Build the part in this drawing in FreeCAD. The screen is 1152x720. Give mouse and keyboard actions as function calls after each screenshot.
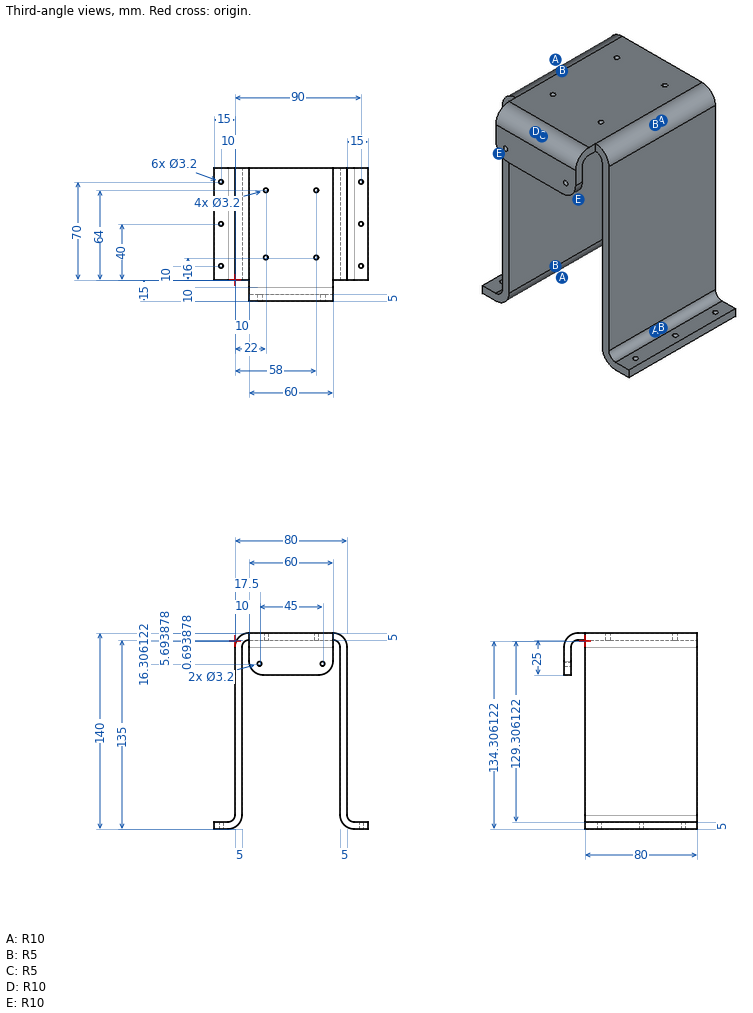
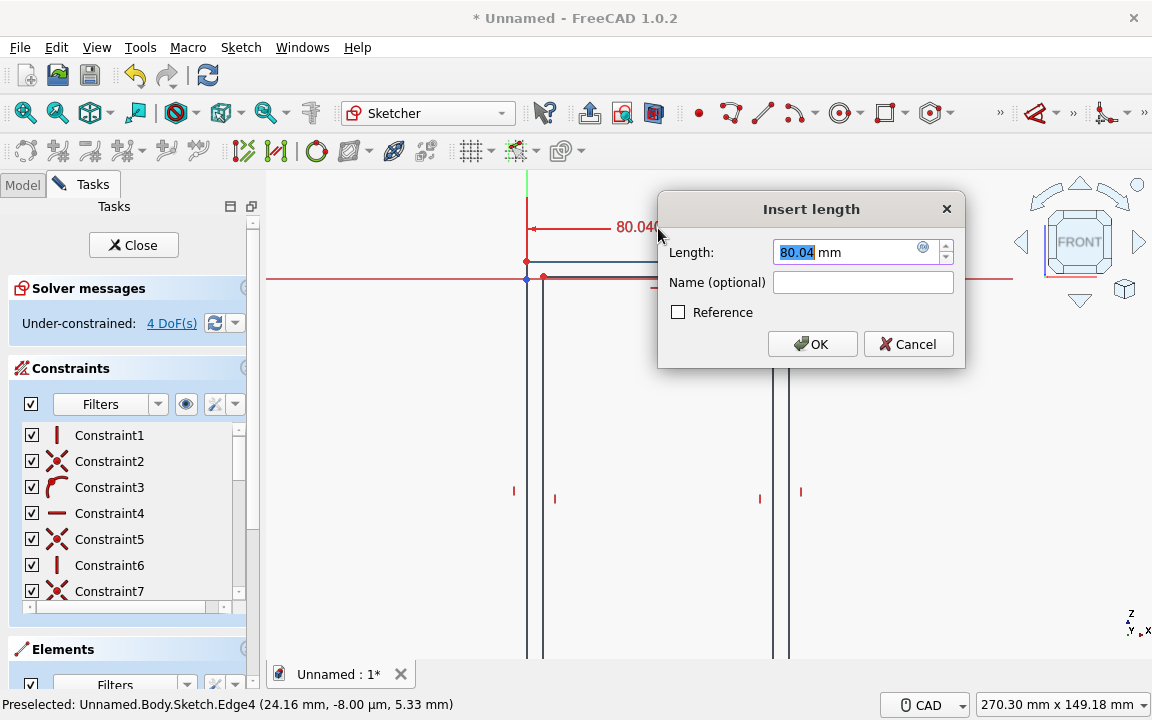
text(80)
key(Return)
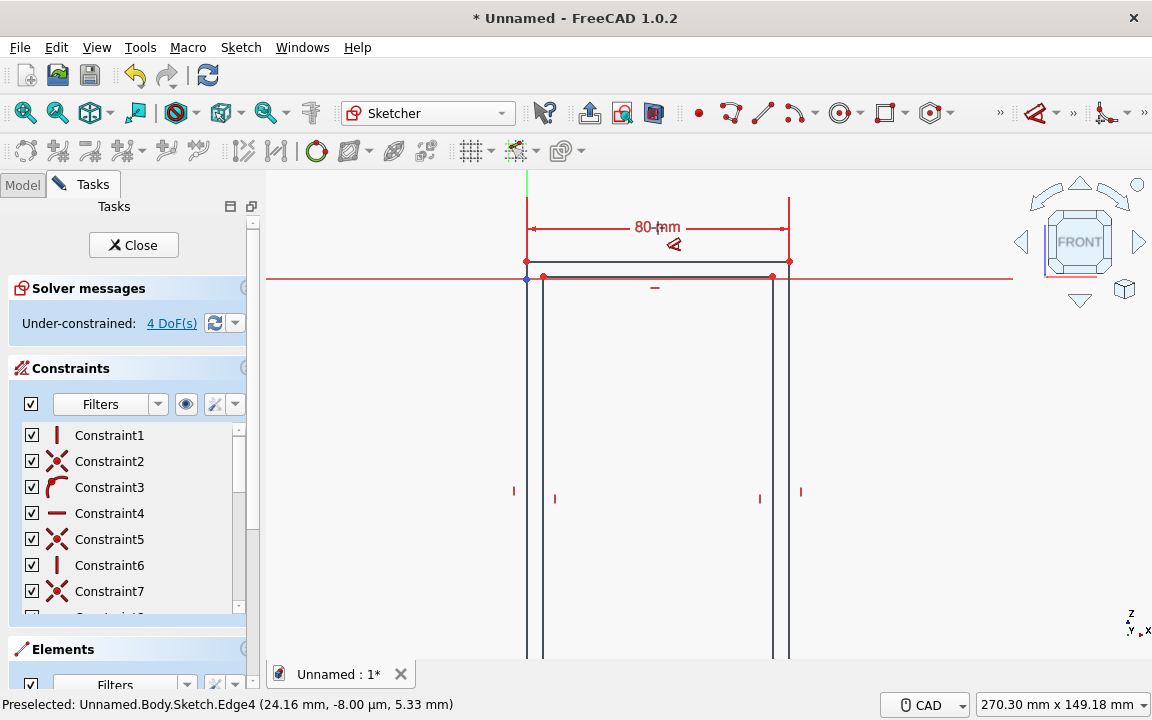
click(543, 410)
click(509, 454)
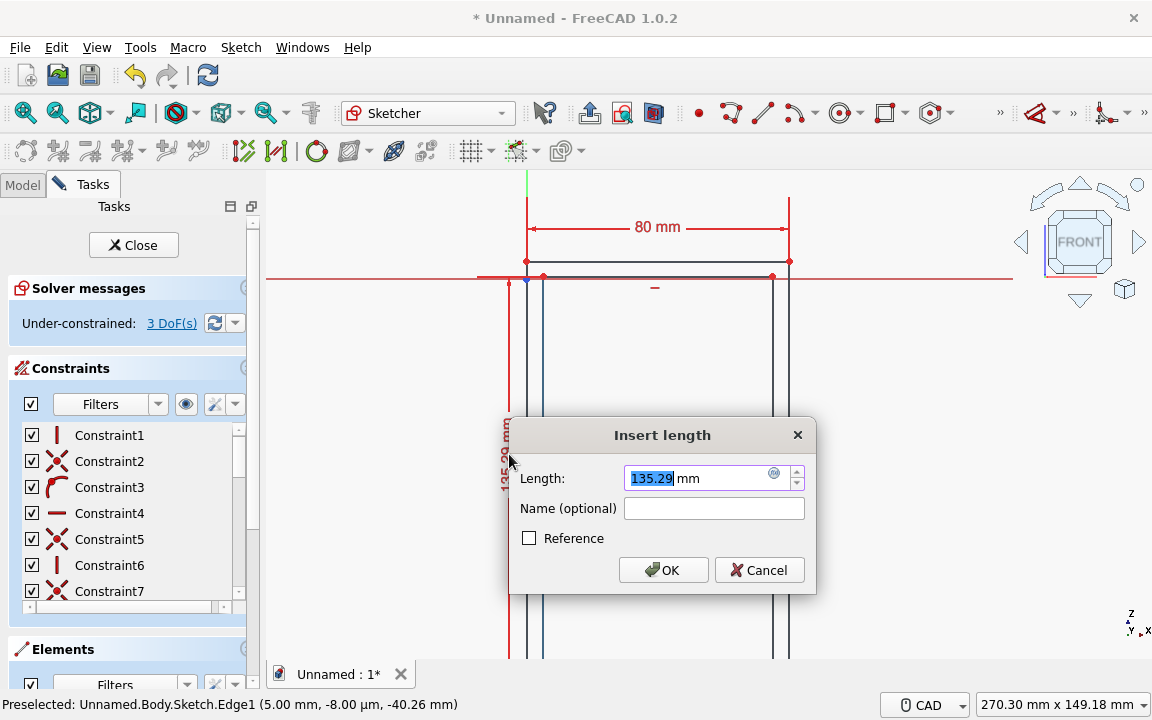
text(135)
key(Return)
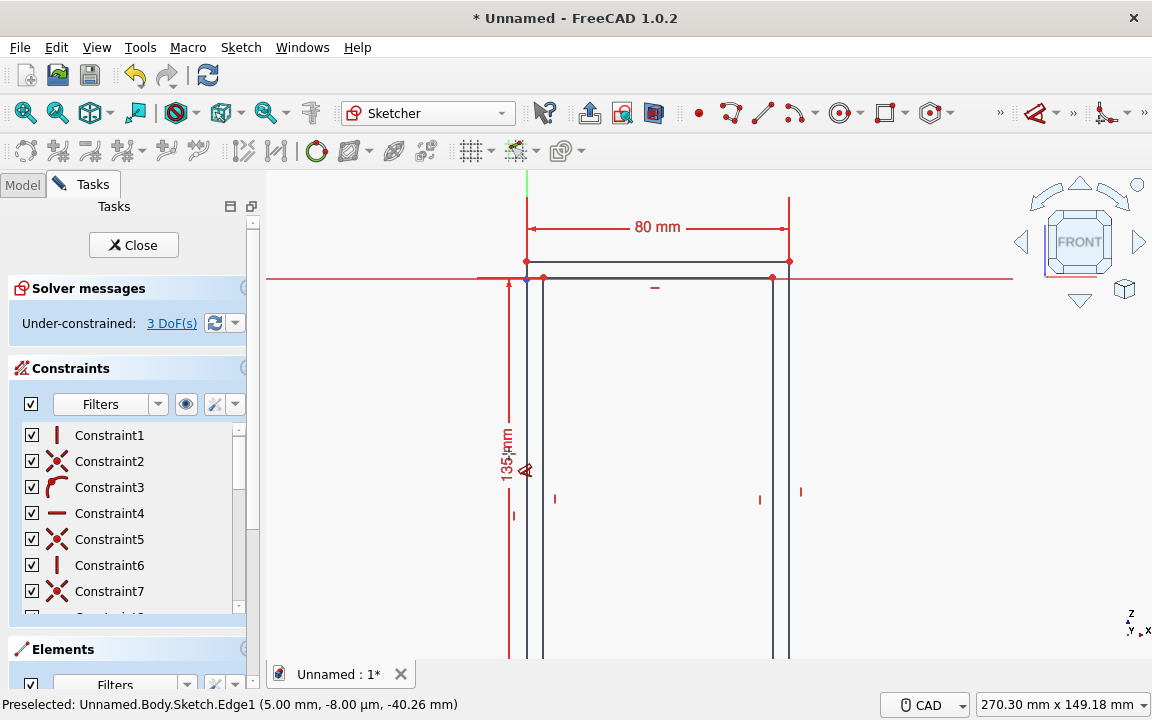
click(527, 583)
click(493, 361)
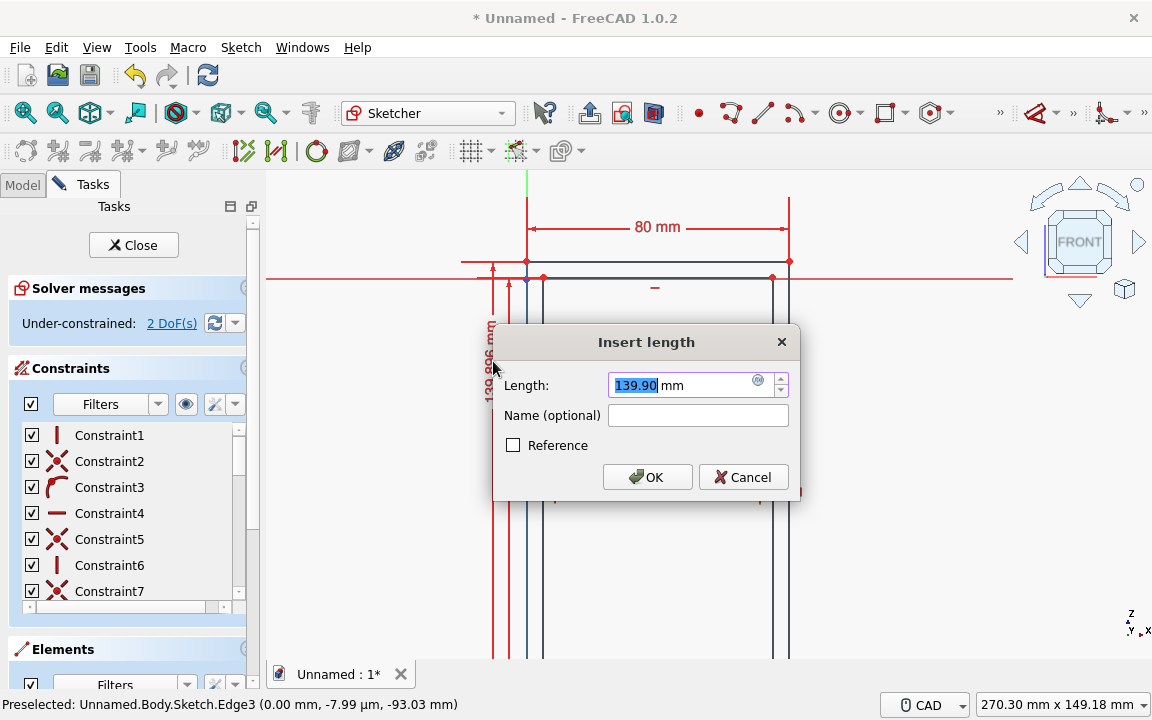
text(140)
key(Return)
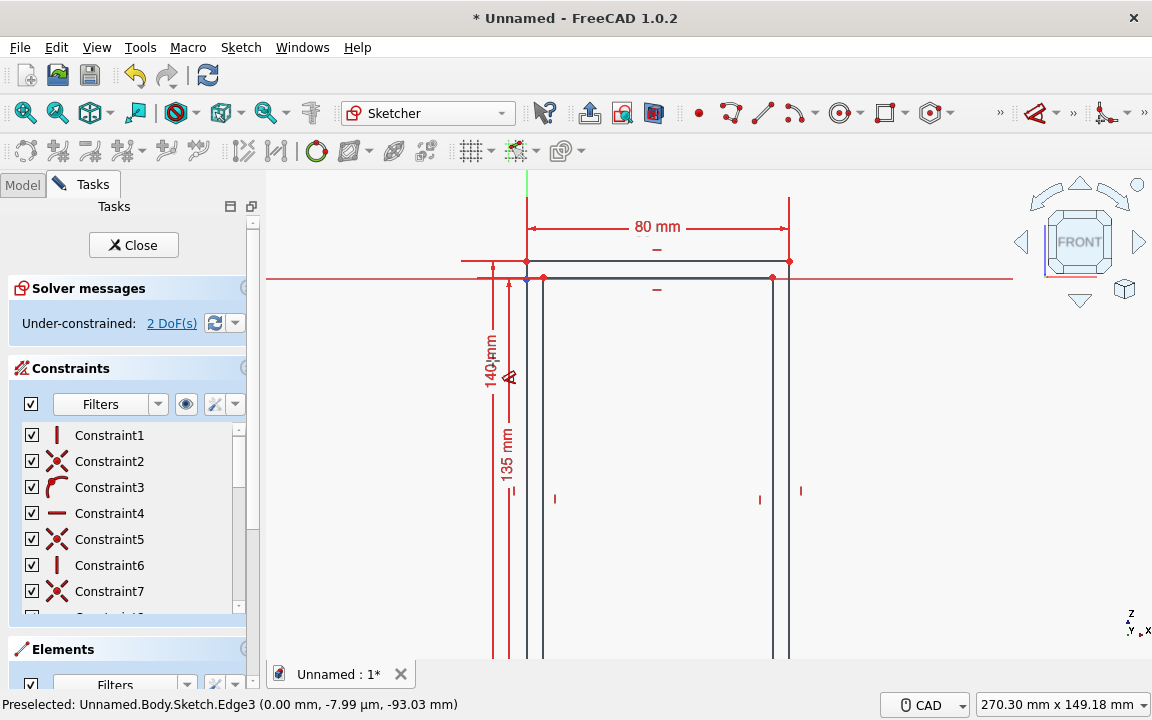
click(789, 399)
click(823, 446)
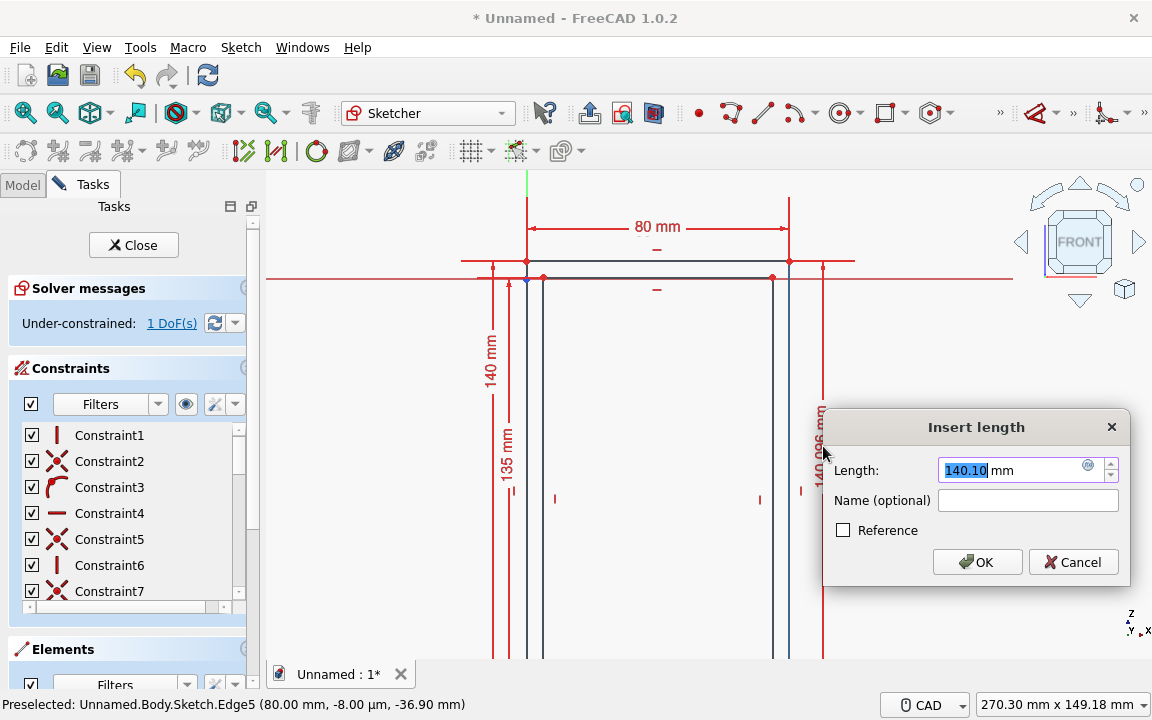
text(140)
key(Return)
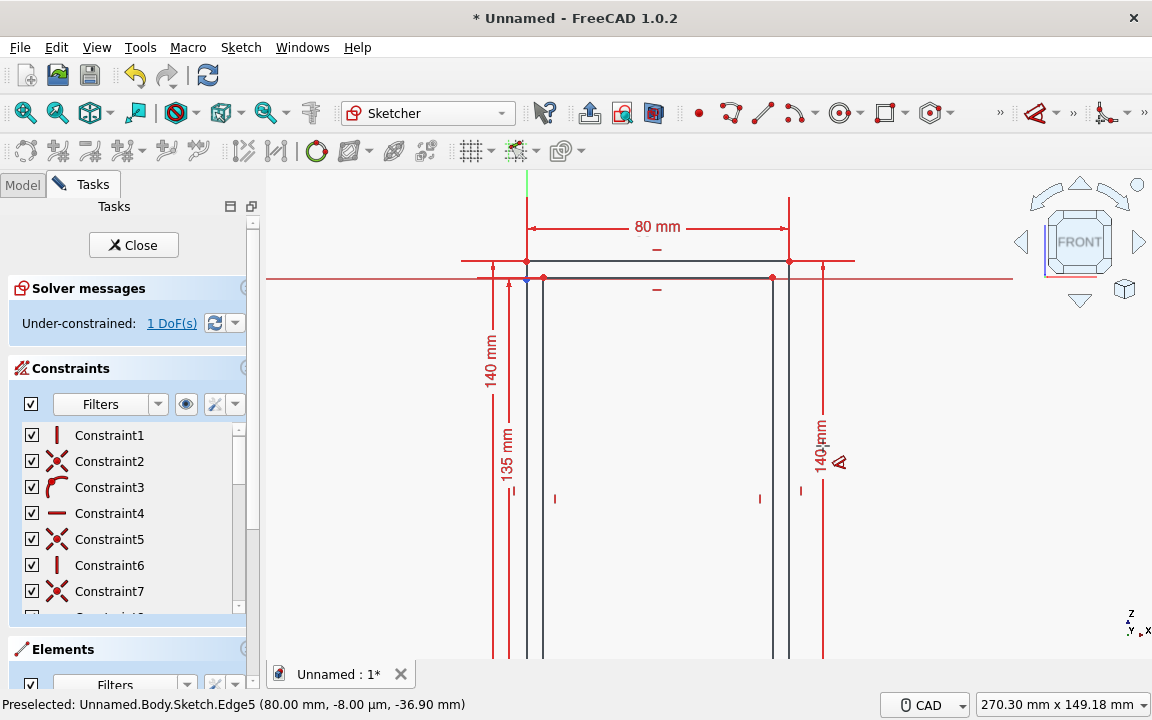
scroll(543, 278, up, 15)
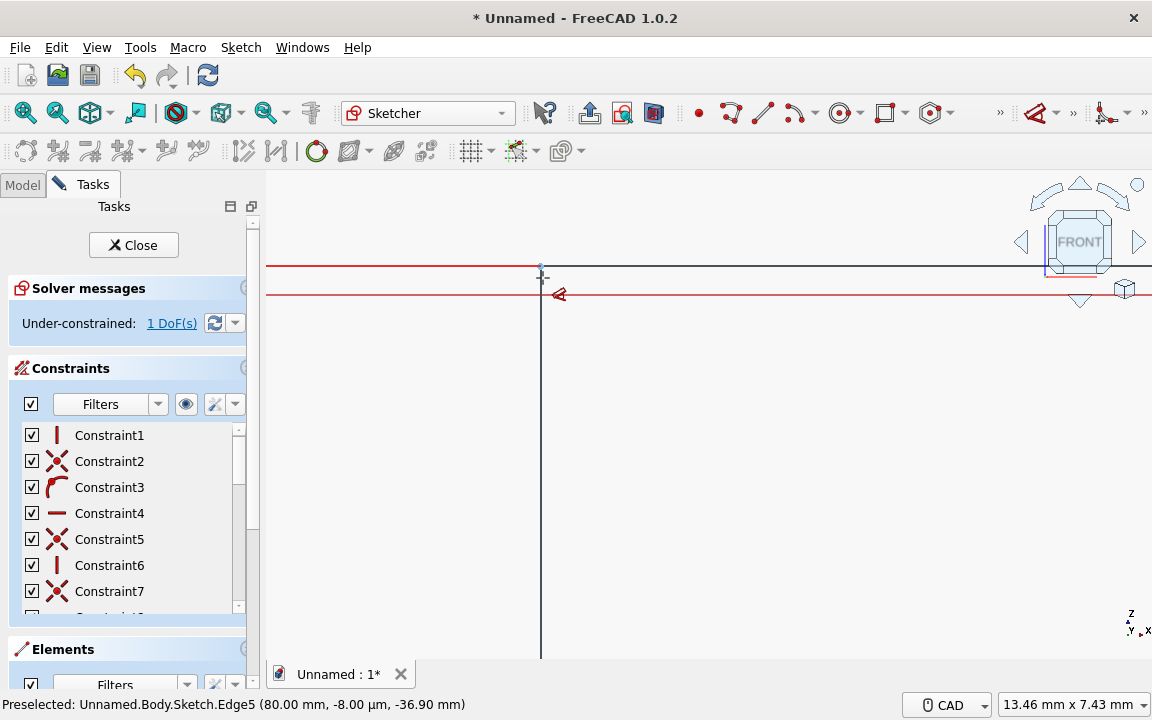
click(541, 266)
click(575, 281)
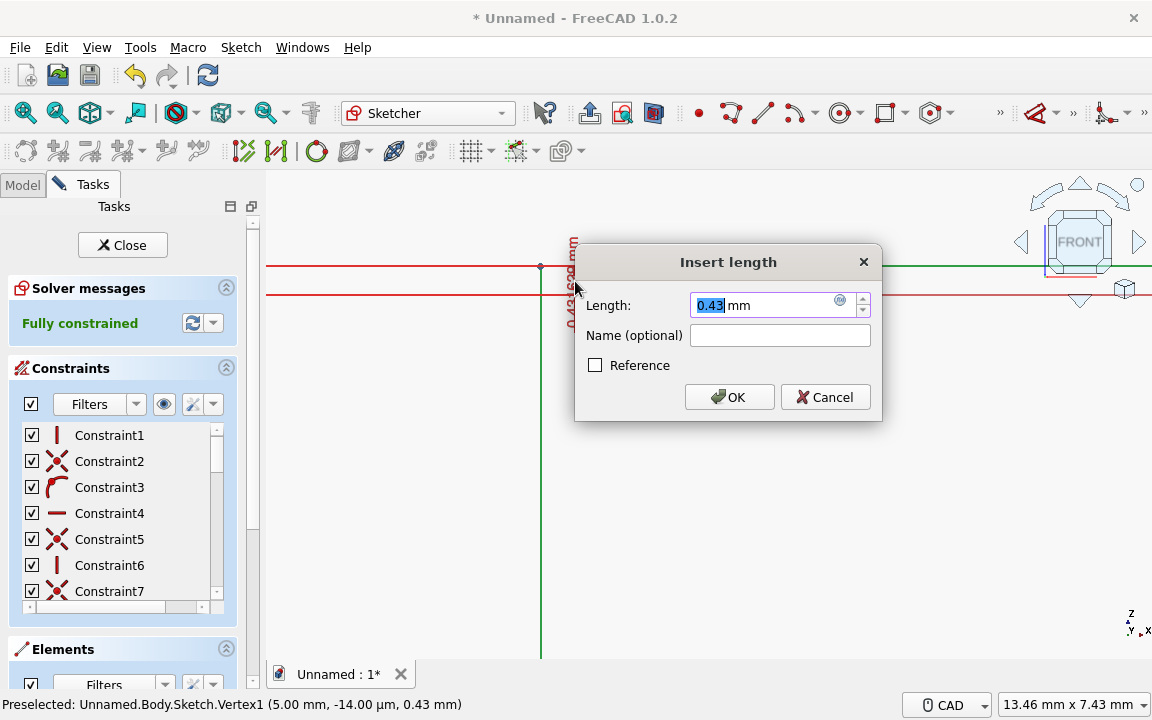
text(0.693878)
key(Return)
key(Escape)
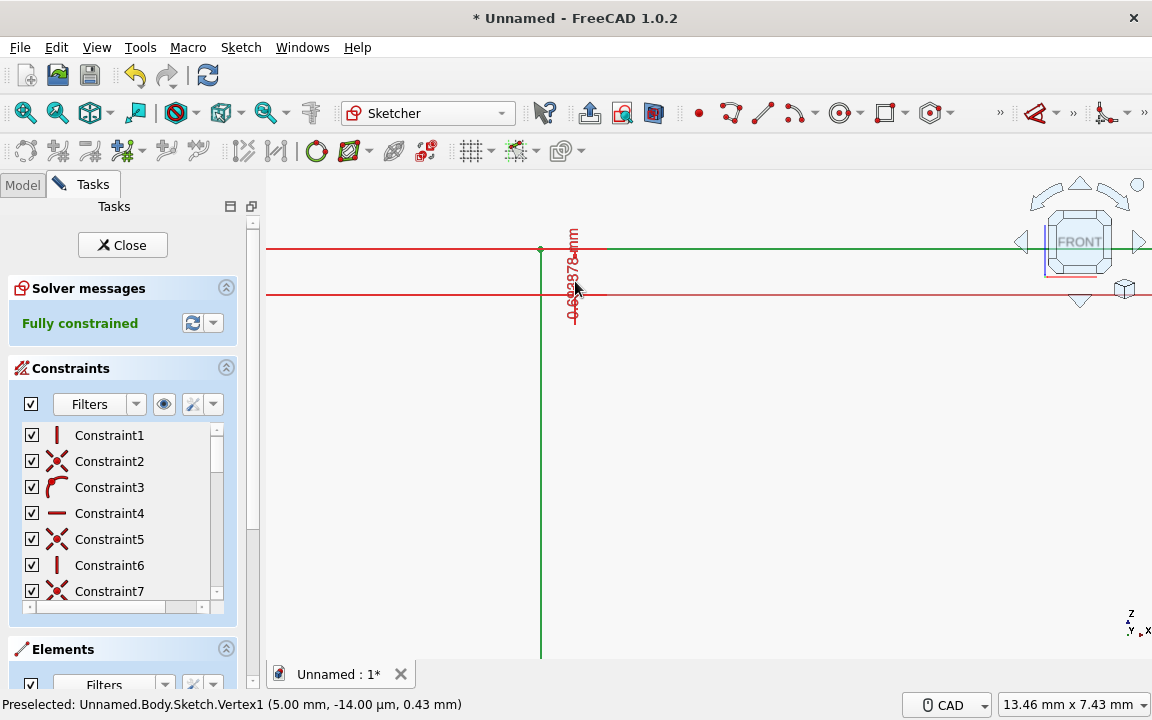
click(123, 245)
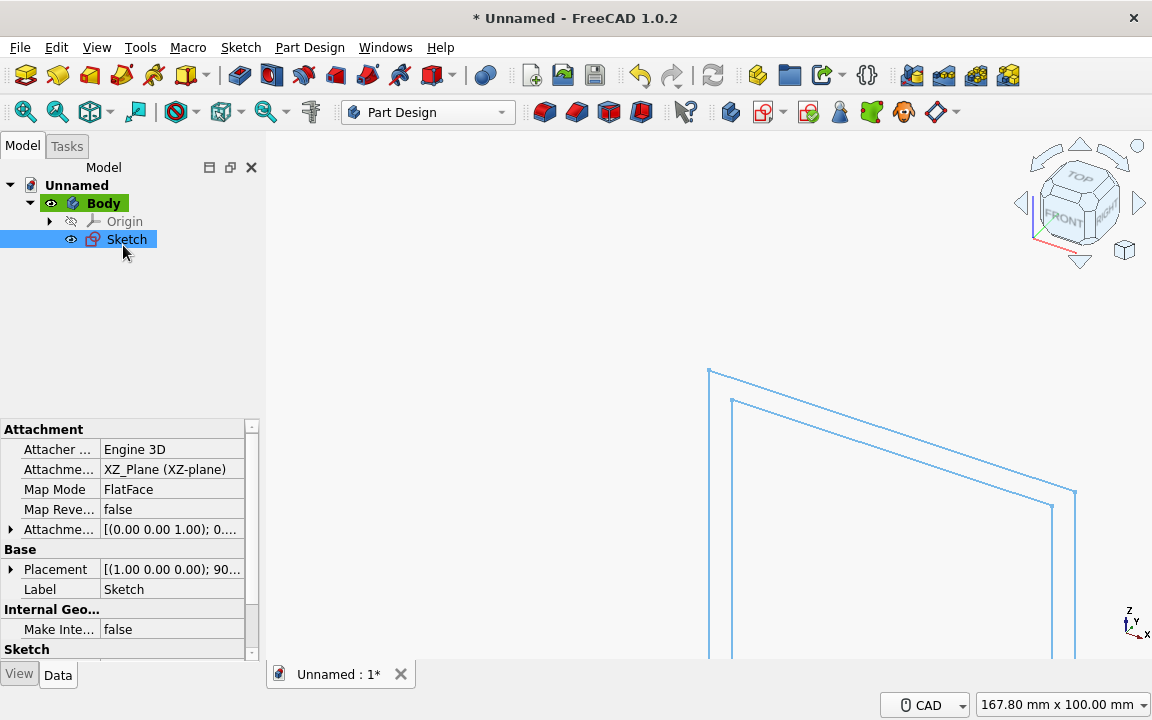
click(26, 76)